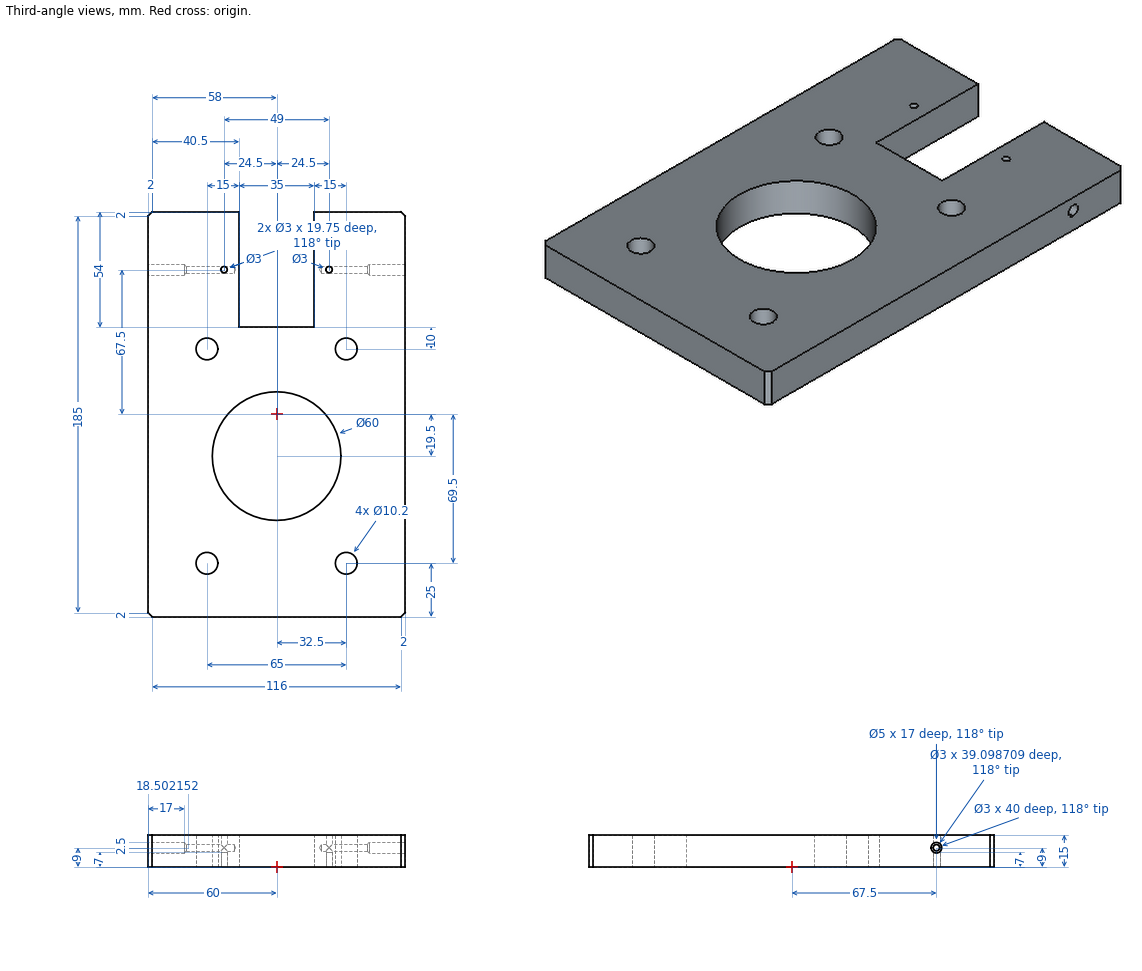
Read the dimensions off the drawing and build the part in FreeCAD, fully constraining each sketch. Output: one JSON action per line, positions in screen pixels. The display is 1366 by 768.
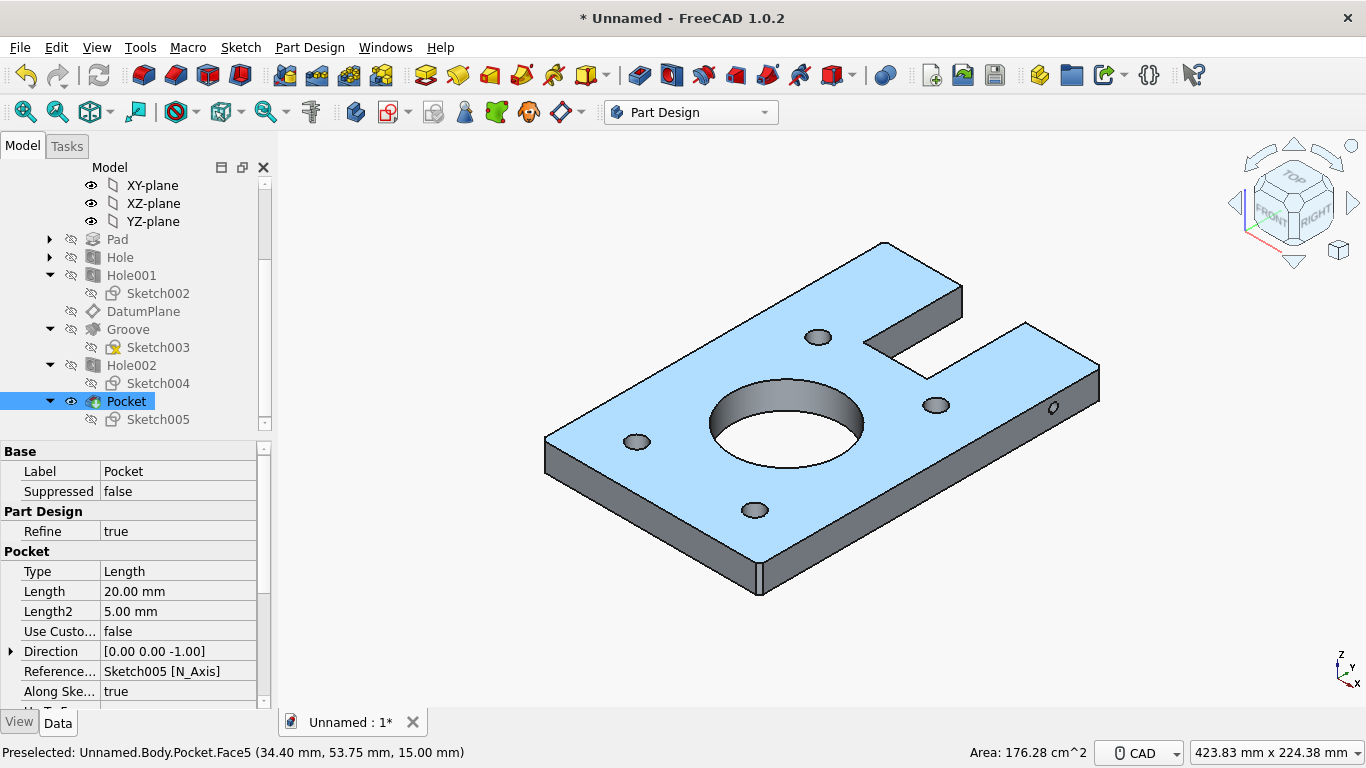
{"action": "left_click", "coordinate": [388, 112]}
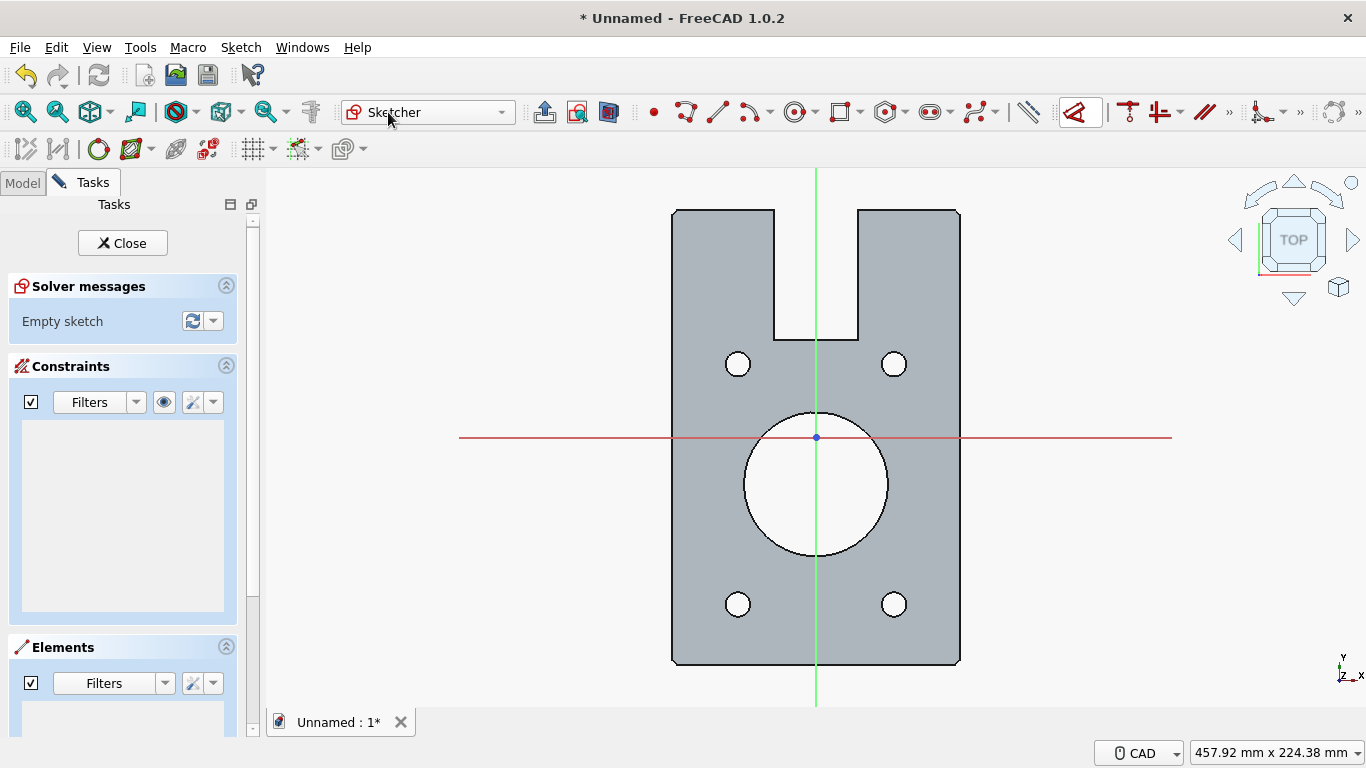
{"action": "scroll", "coordinate": [872, 287], "scroll_direction": "up", "scroll_amount": 4}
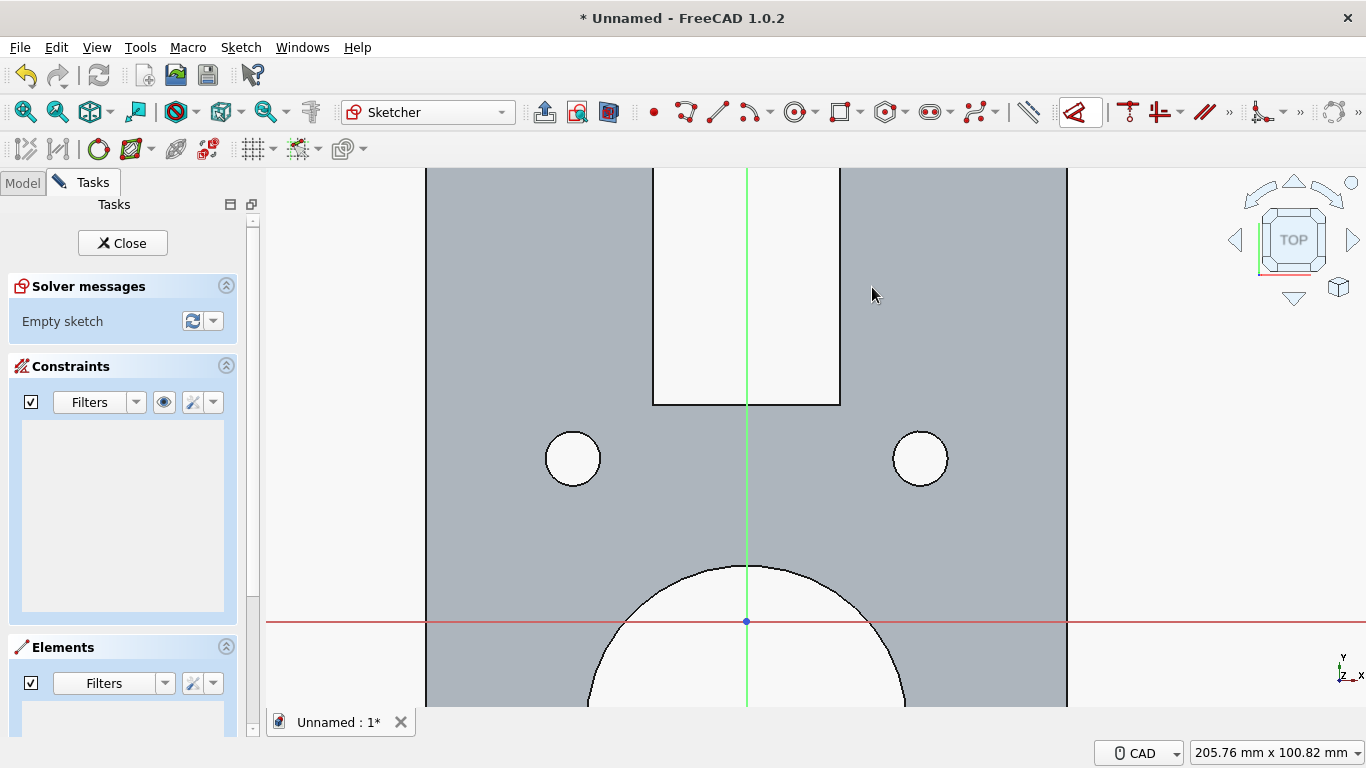
{"action": "left_click", "coordinate": [796, 112]}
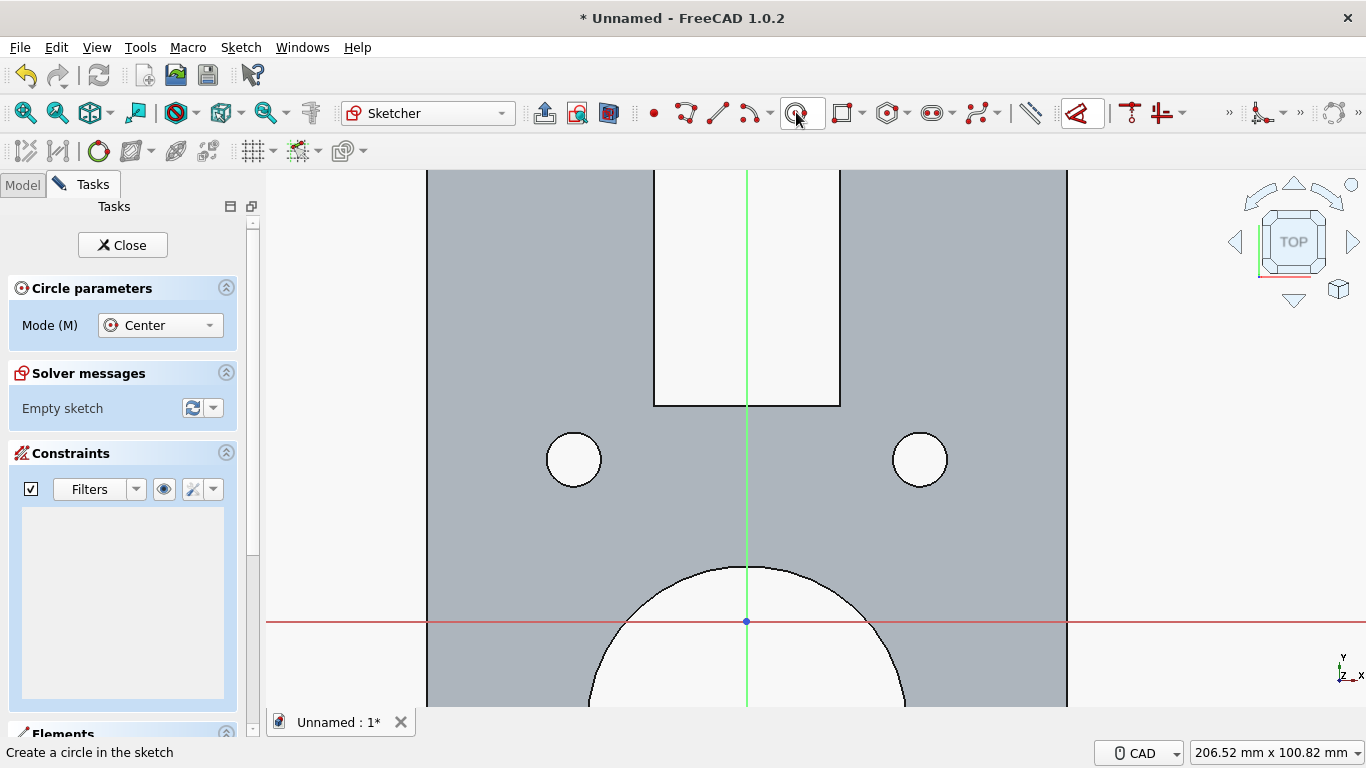
{"action": "scroll", "coordinate": [616, 262], "scroll_direction": "up", "scroll_amount": 6}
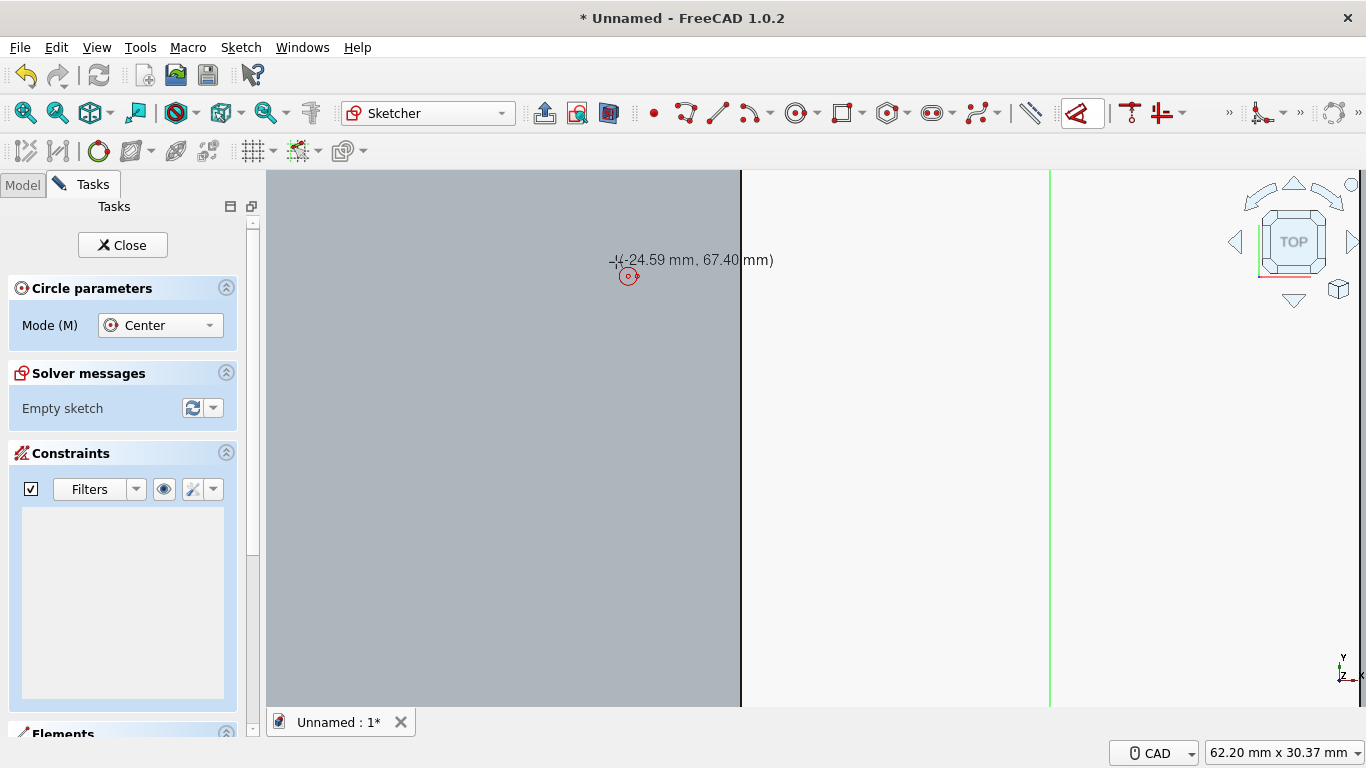
{"action": "left_click", "coordinate": [617, 263]}
{"action": "mouse_move", "coordinate": [636, 244]}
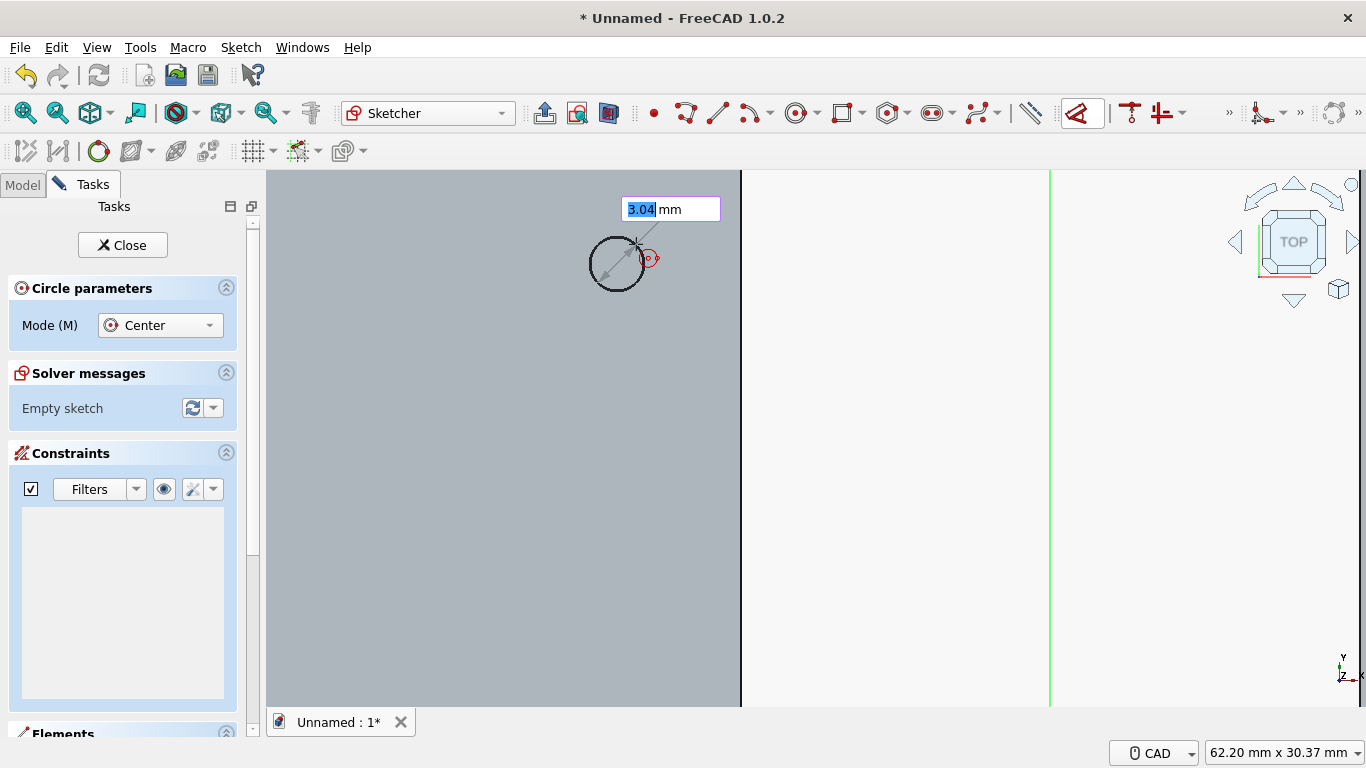
{"action": "type", "text": "3"}
{"action": "key", "text": "Return"}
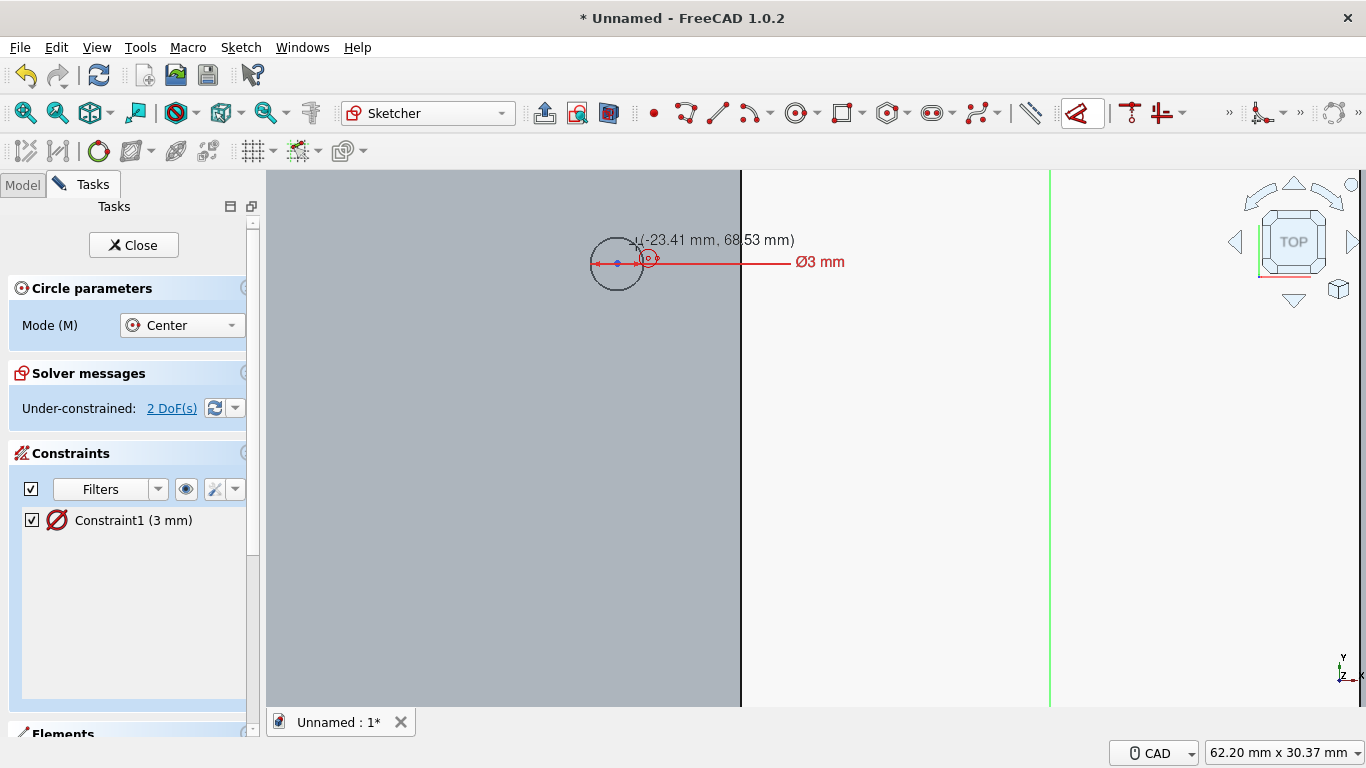
{"action": "scroll", "coordinate": [617, 263], "scroll_direction": "down", "scroll_amount": 6}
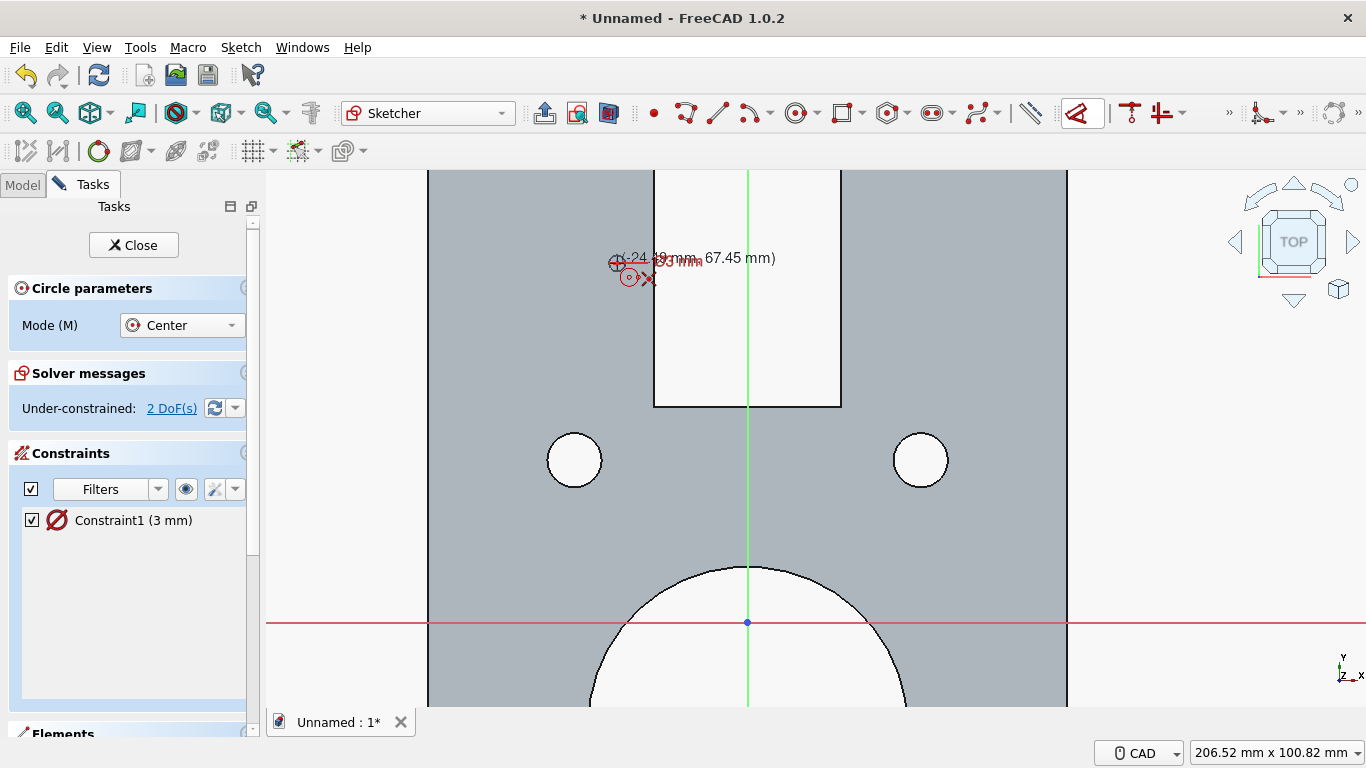
{"action": "scroll", "coordinate": [878, 263], "scroll_direction": "up", "scroll_amount": 6}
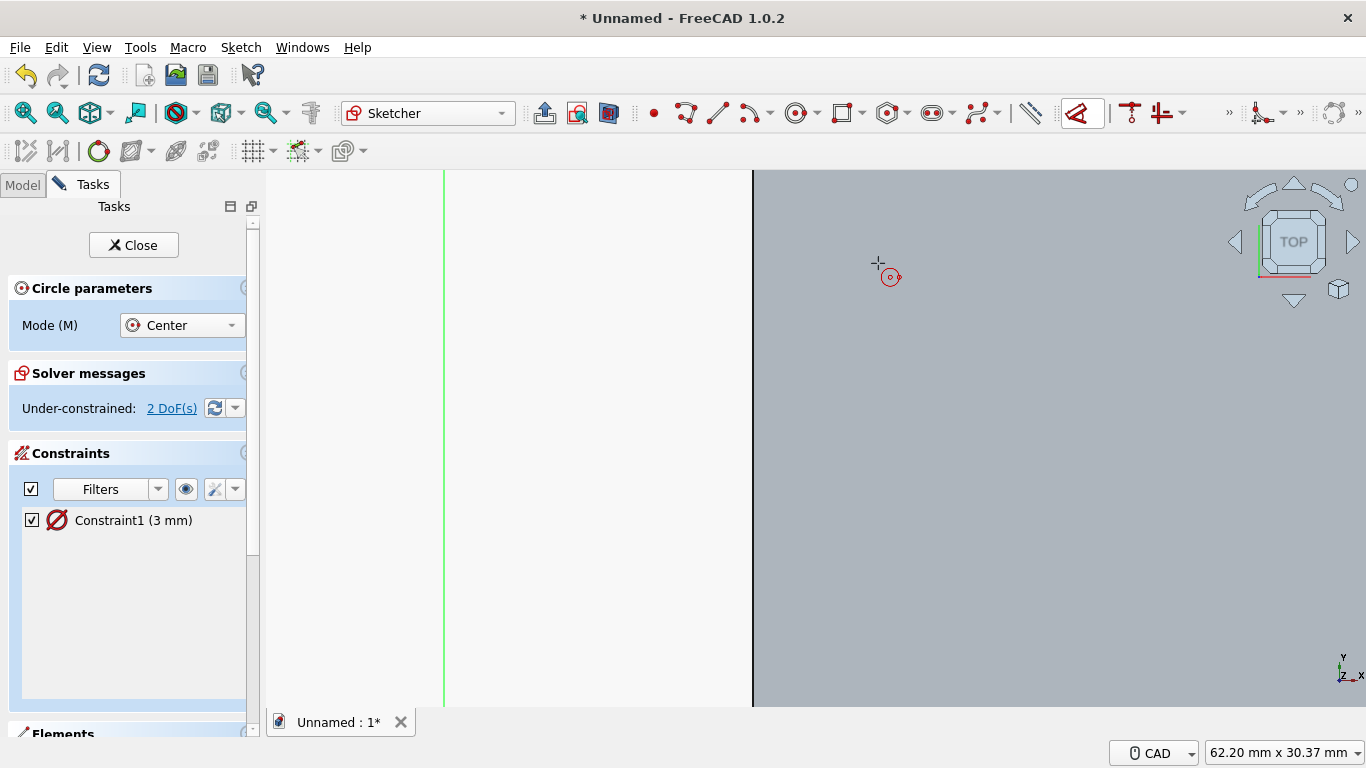
{"action": "left_click", "coordinate": [877, 263]}
{"action": "mouse_move", "coordinate": [896, 244]}